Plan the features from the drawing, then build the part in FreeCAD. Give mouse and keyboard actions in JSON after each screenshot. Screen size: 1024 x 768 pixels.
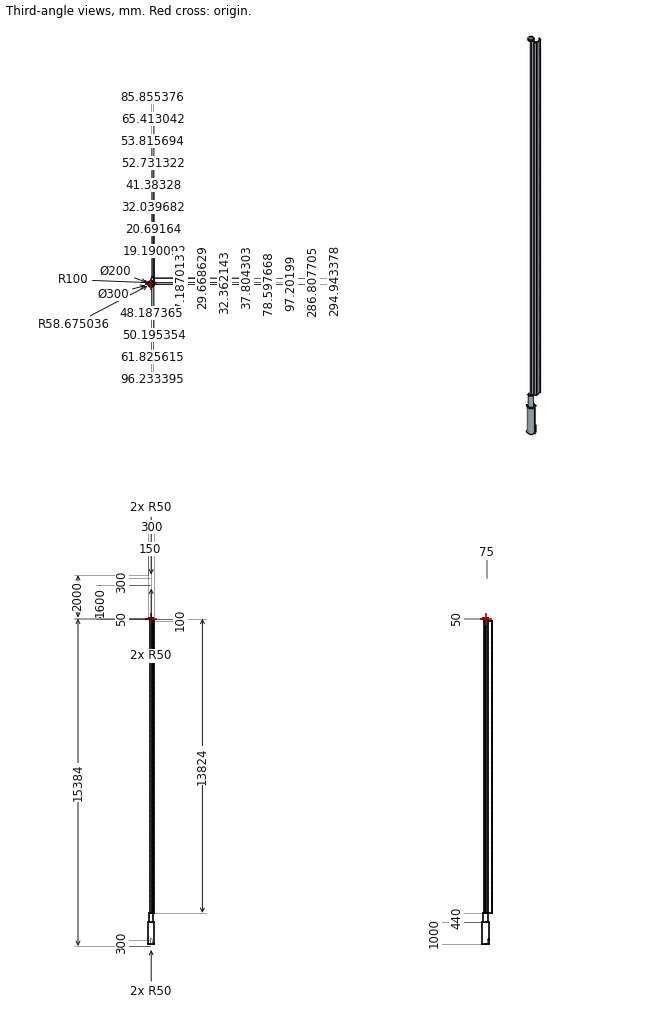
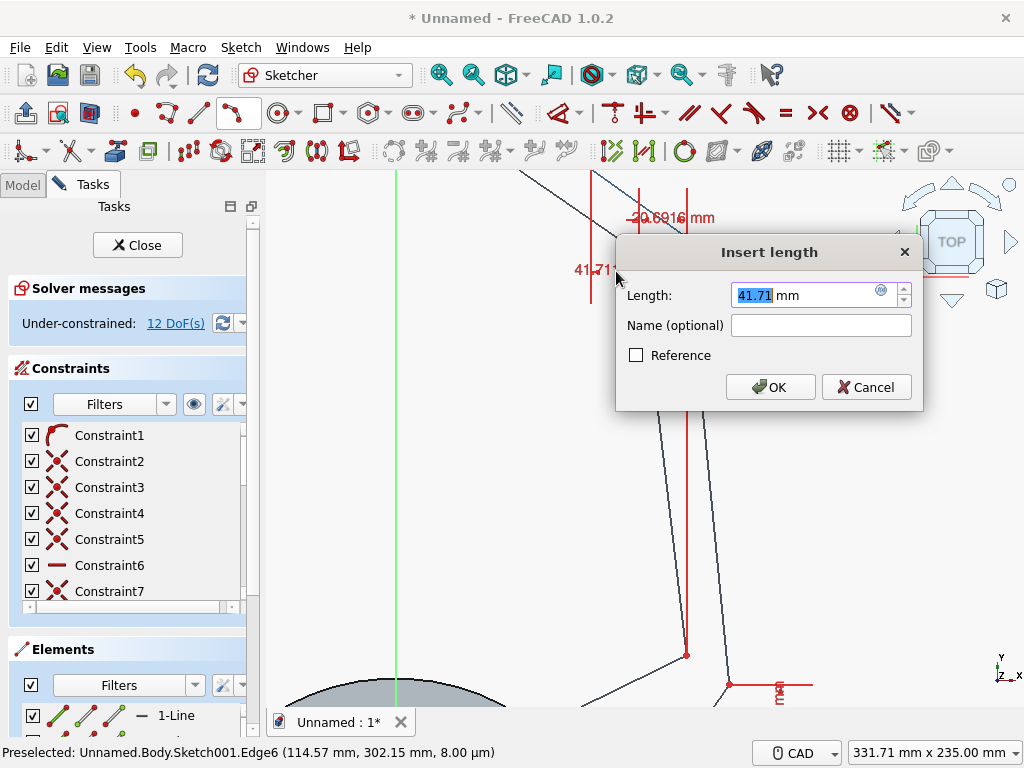
{"action": "type", "text": "41.38328"}
{"action": "key", "text": "Return"}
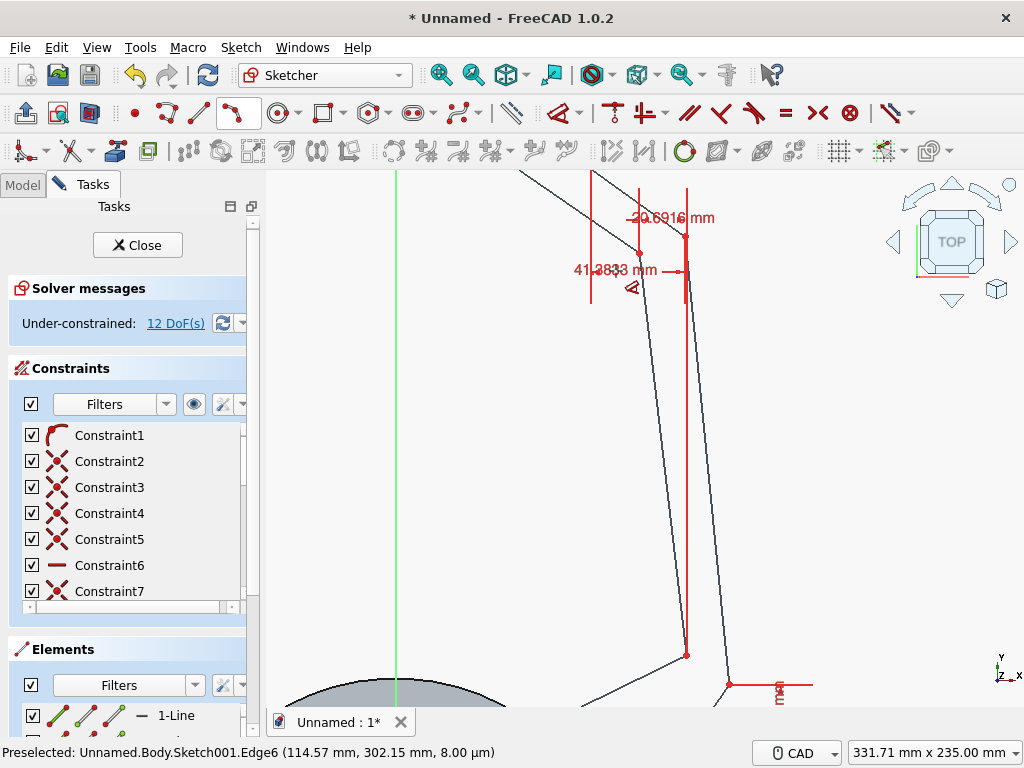
{"action": "scroll", "coordinate": [636, 328], "scroll_direction": "down", "scroll_amount": 4}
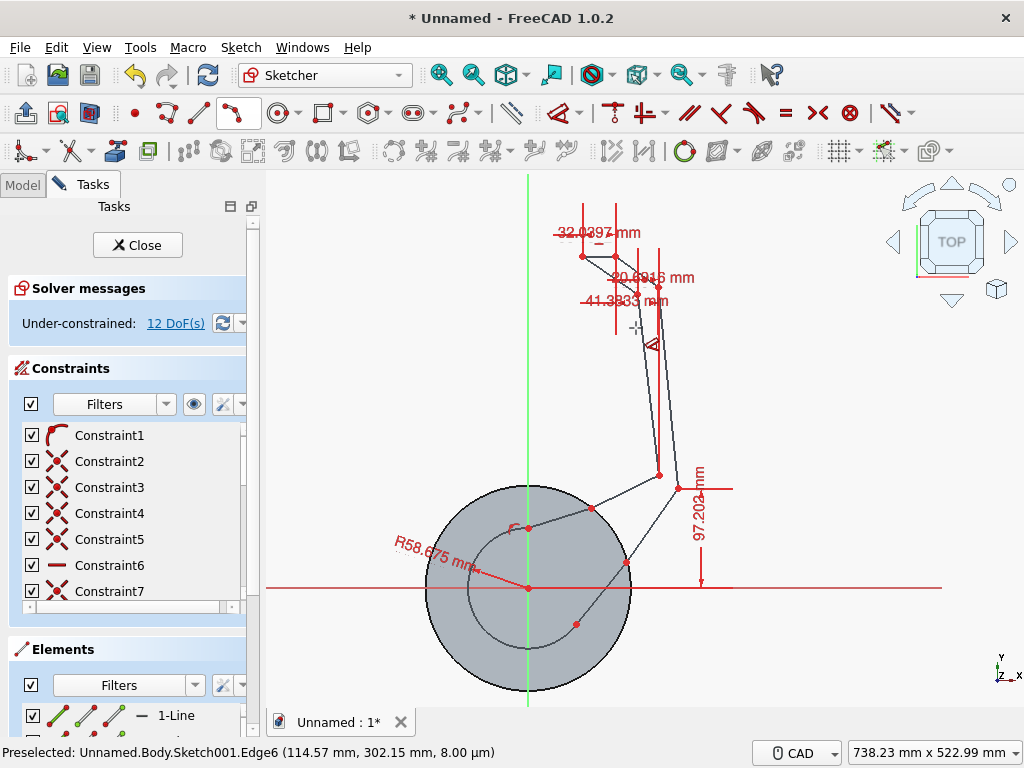
{"action": "left_click", "coordinate": [591, 508]}
{"action": "left_click", "coordinate": [560, 622]}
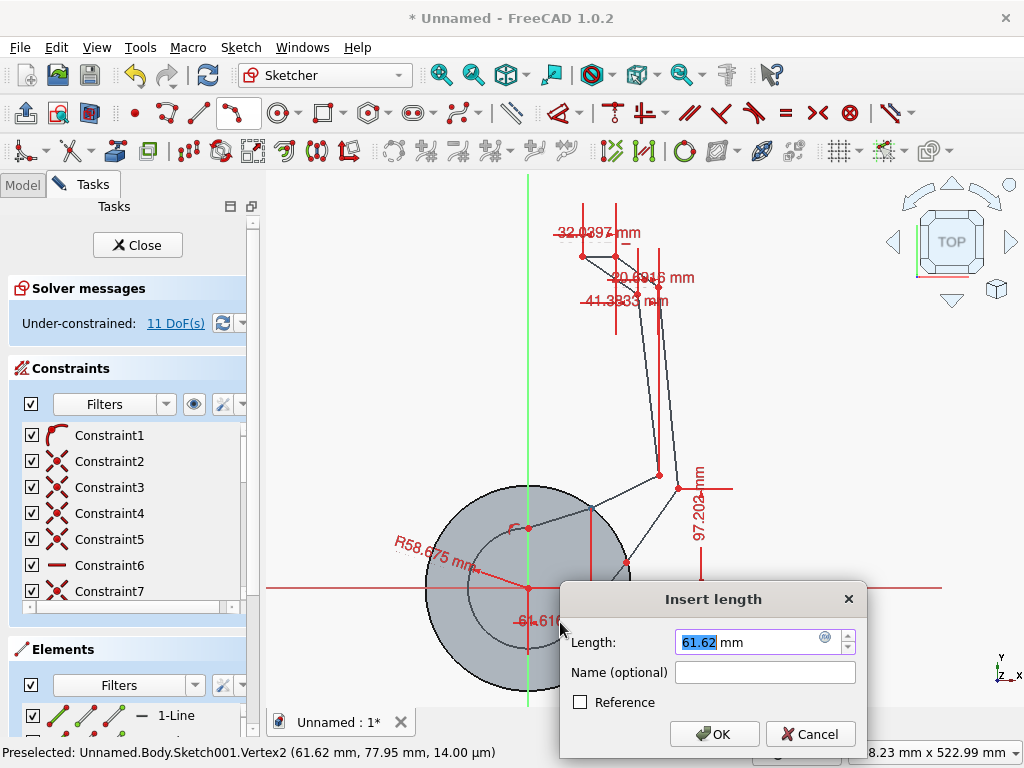
{"action": "type", "text": "61.825615"}
{"action": "key", "text": "Return"}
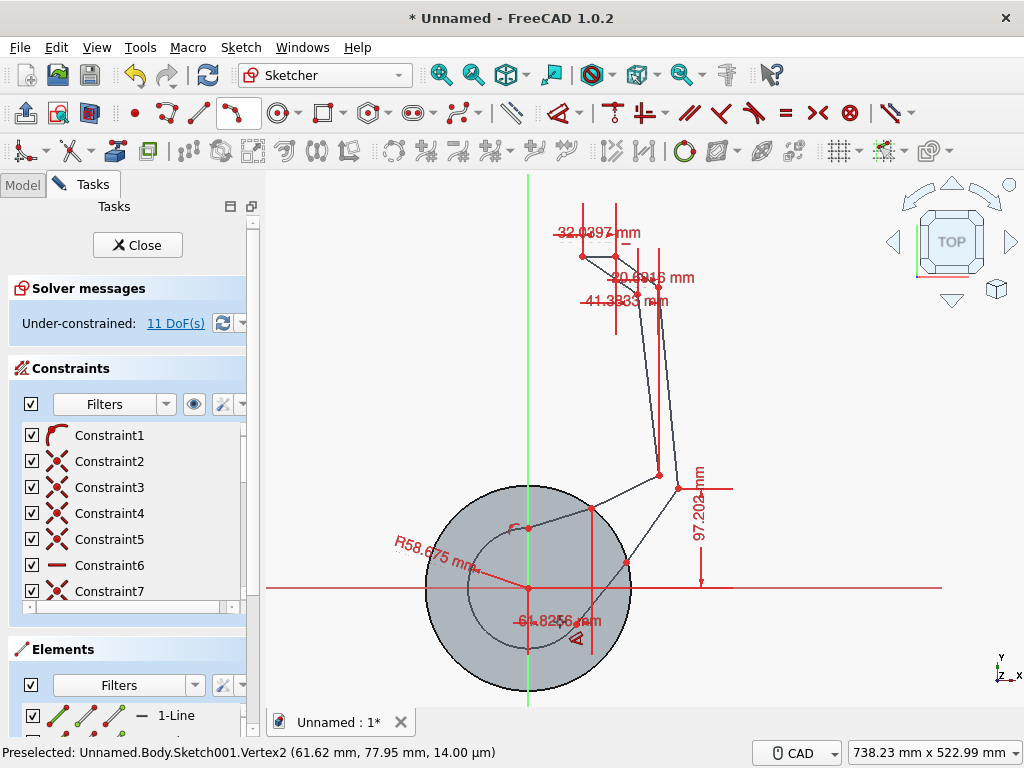
{"action": "left_click", "coordinate": [592, 508]}
{"action": "left_click", "coordinate": [494, 520]}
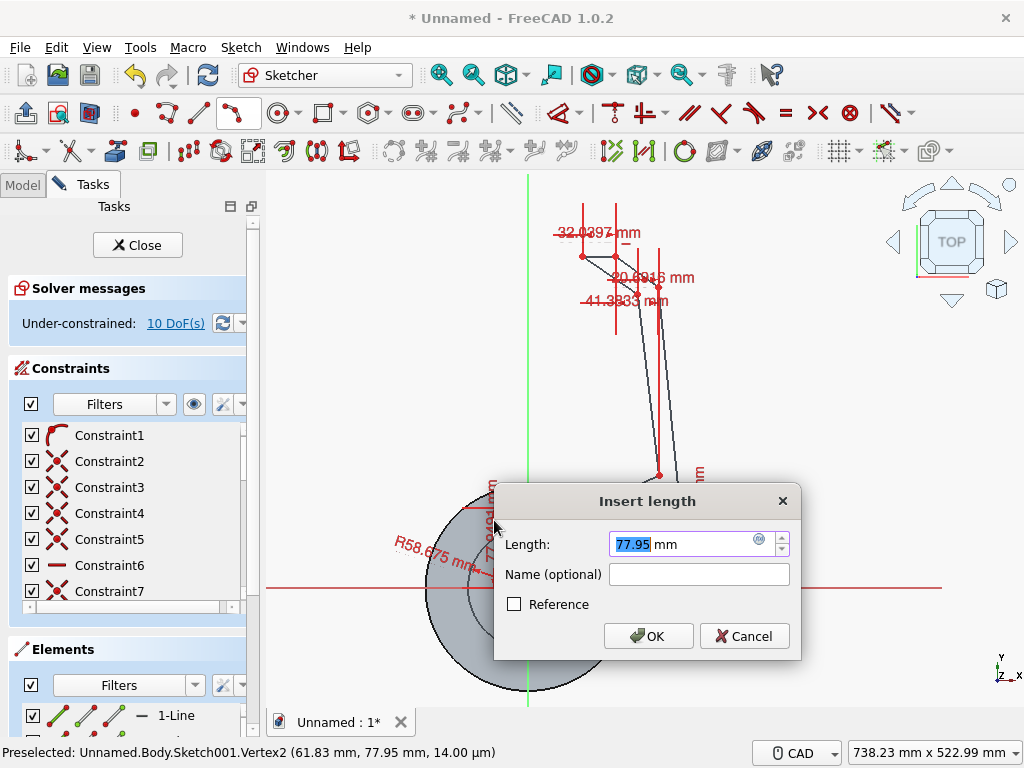
{"action": "type", "text": "78.597668"}
{"action": "key", "text": "Return"}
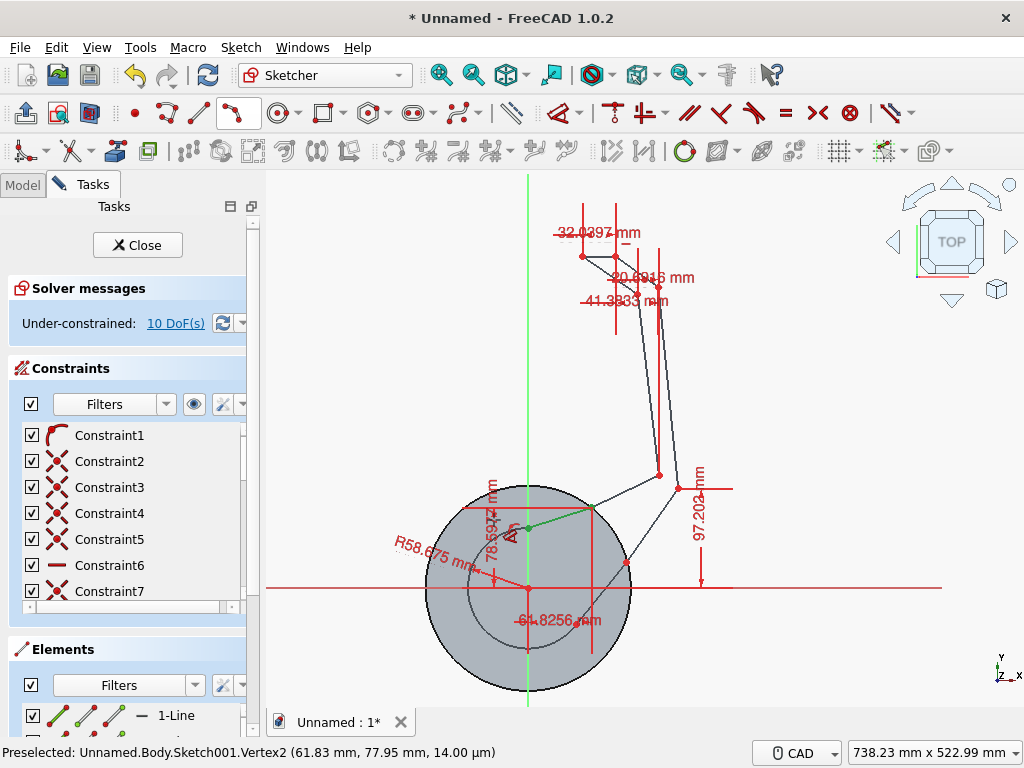
{"action": "left_click", "coordinate": [583, 257]}
{"action": "left_click", "coordinate": [556, 199]}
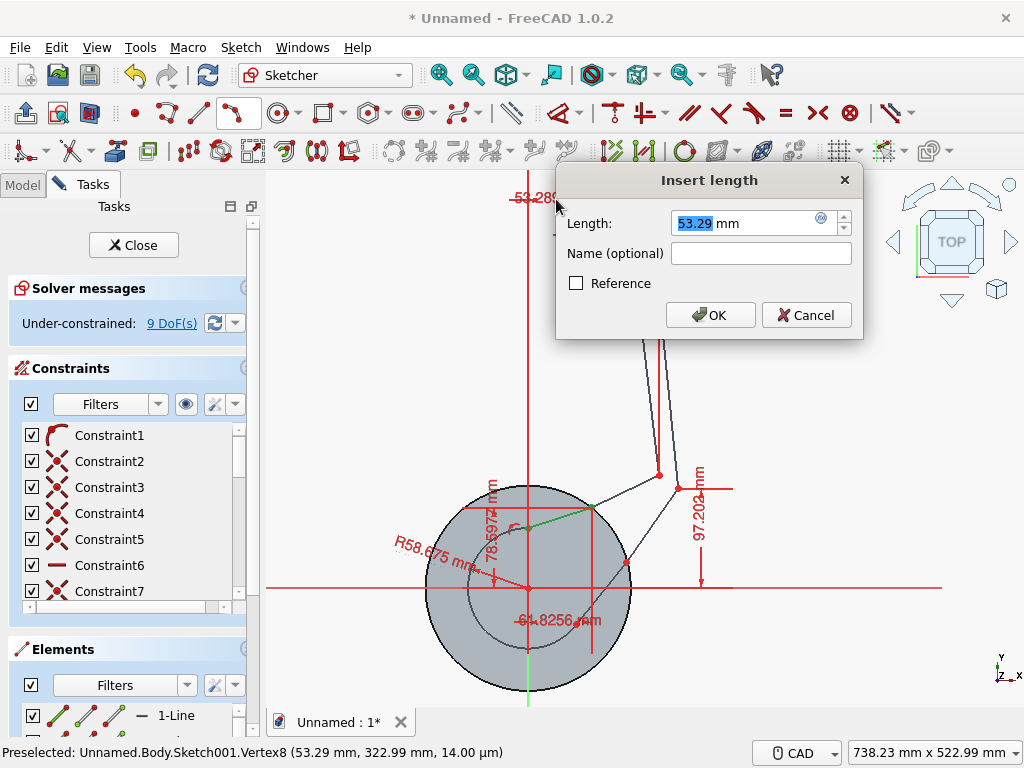
{"action": "type", "text": "53.815694"}
{"action": "key", "text": "Return"}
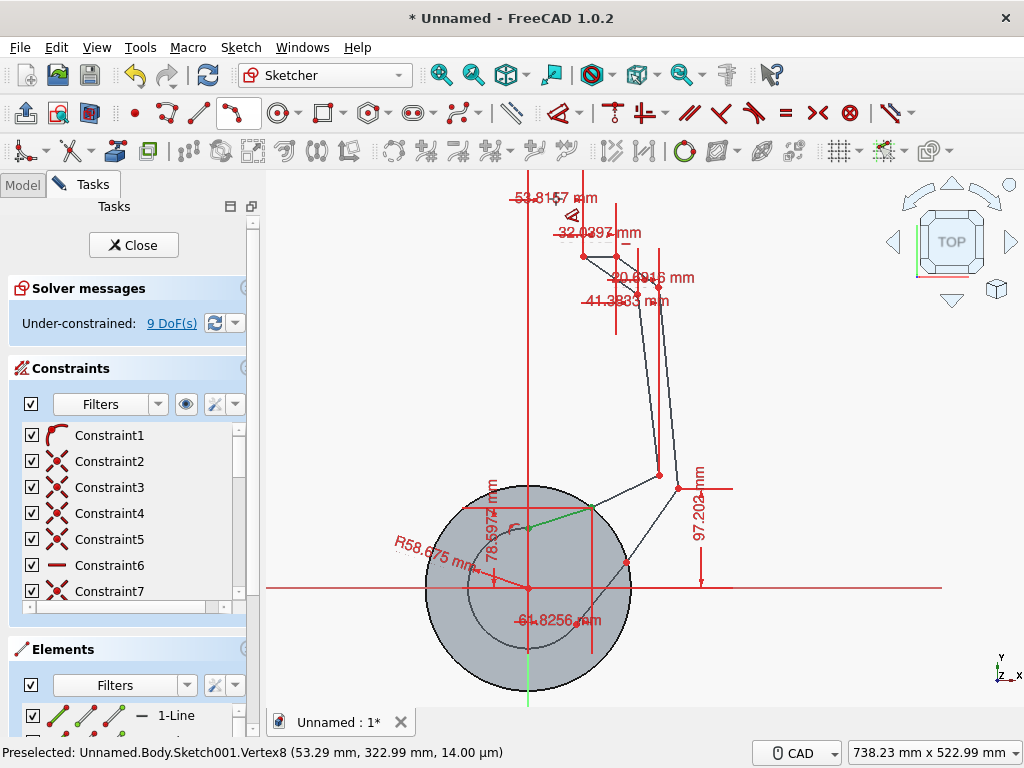
{"action": "left_click", "coordinate": [627, 562]}
{"action": "left_click", "coordinate": [578, 528]}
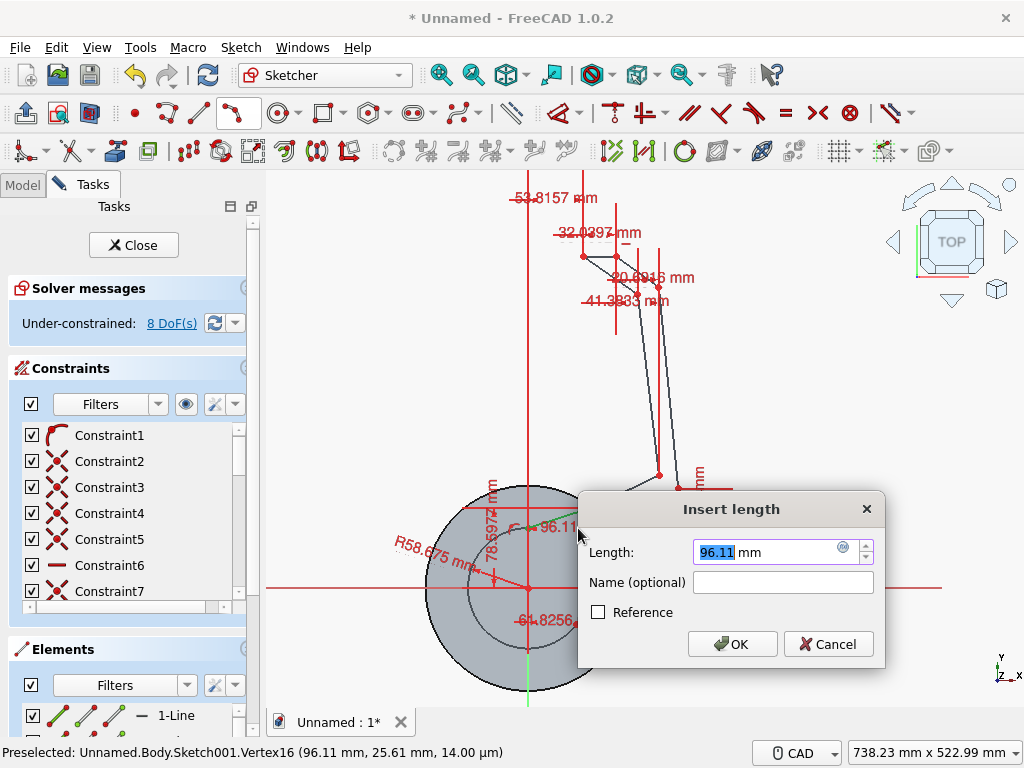
{"action": "type", "text": "96.233395"}
{"action": "key", "text": "Return"}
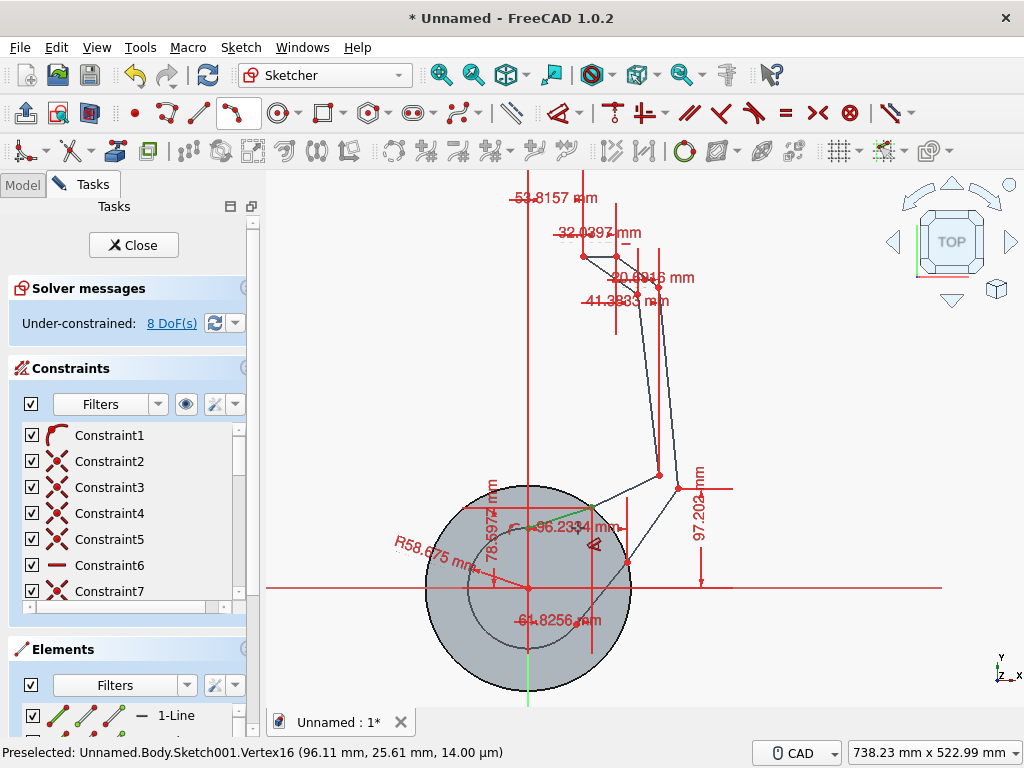
{"action": "scroll", "coordinate": [627, 562], "scroll_direction": "up", "scroll_amount": 2}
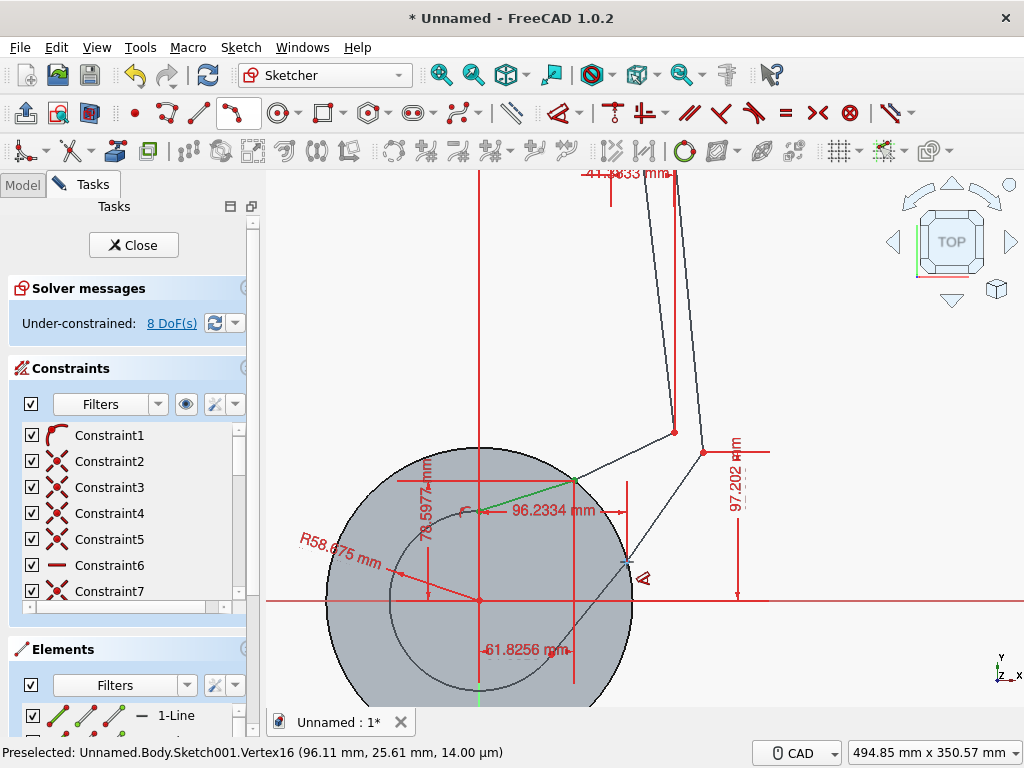
{"action": "left_click", "coordinate": [627, 562]}
{"action": "left_click", "coordinate": [661, 581]}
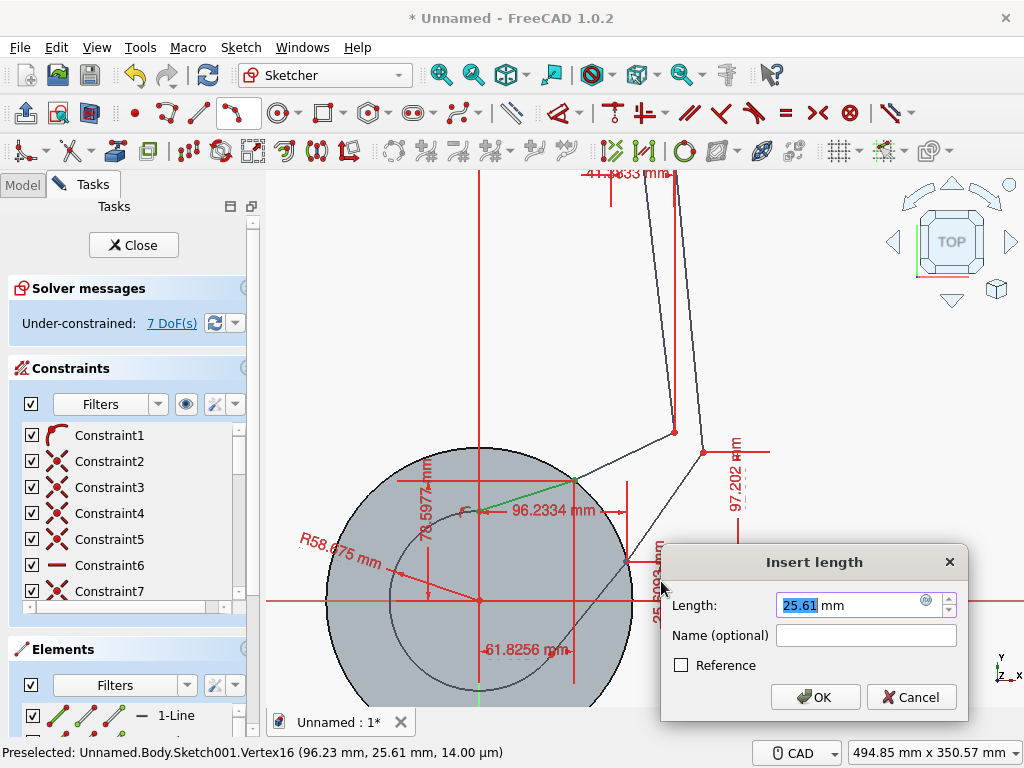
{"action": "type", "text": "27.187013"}
{"action": "key", "text": "Return"}